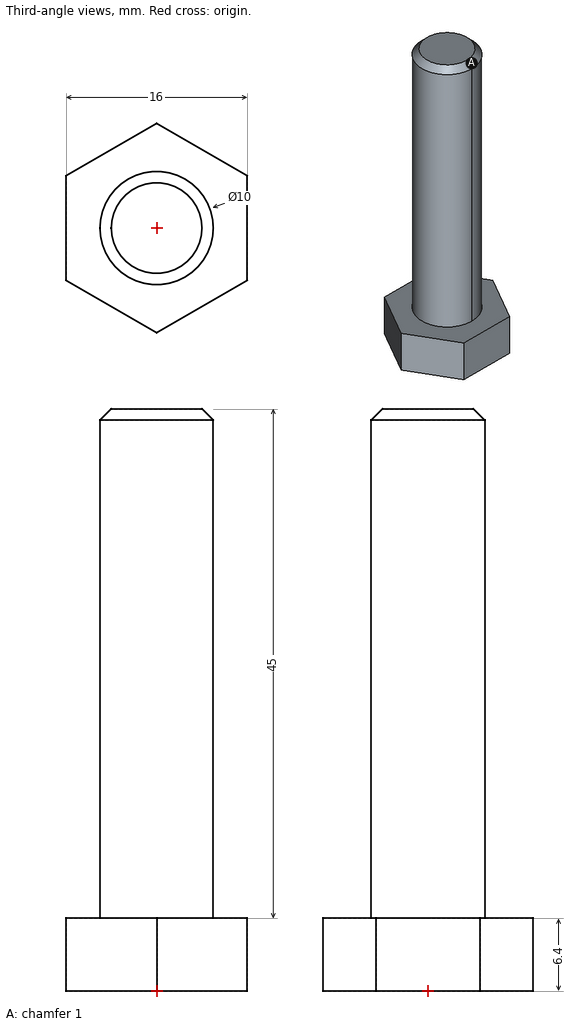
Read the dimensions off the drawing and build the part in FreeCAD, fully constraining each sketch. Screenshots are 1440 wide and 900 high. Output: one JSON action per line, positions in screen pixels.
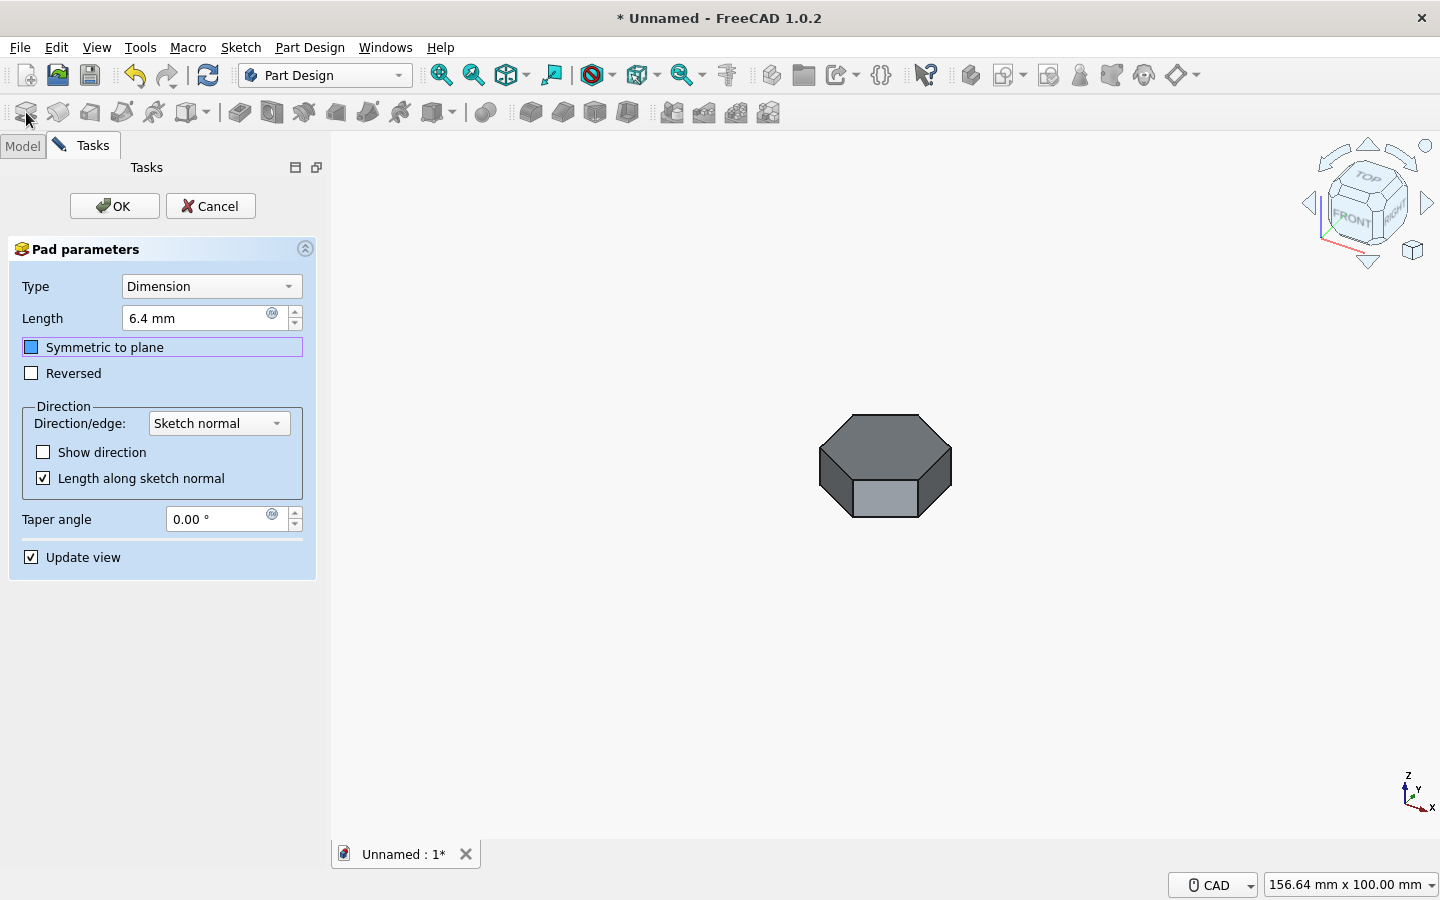
{"action": "left_click", "coordinate": [115, 206]}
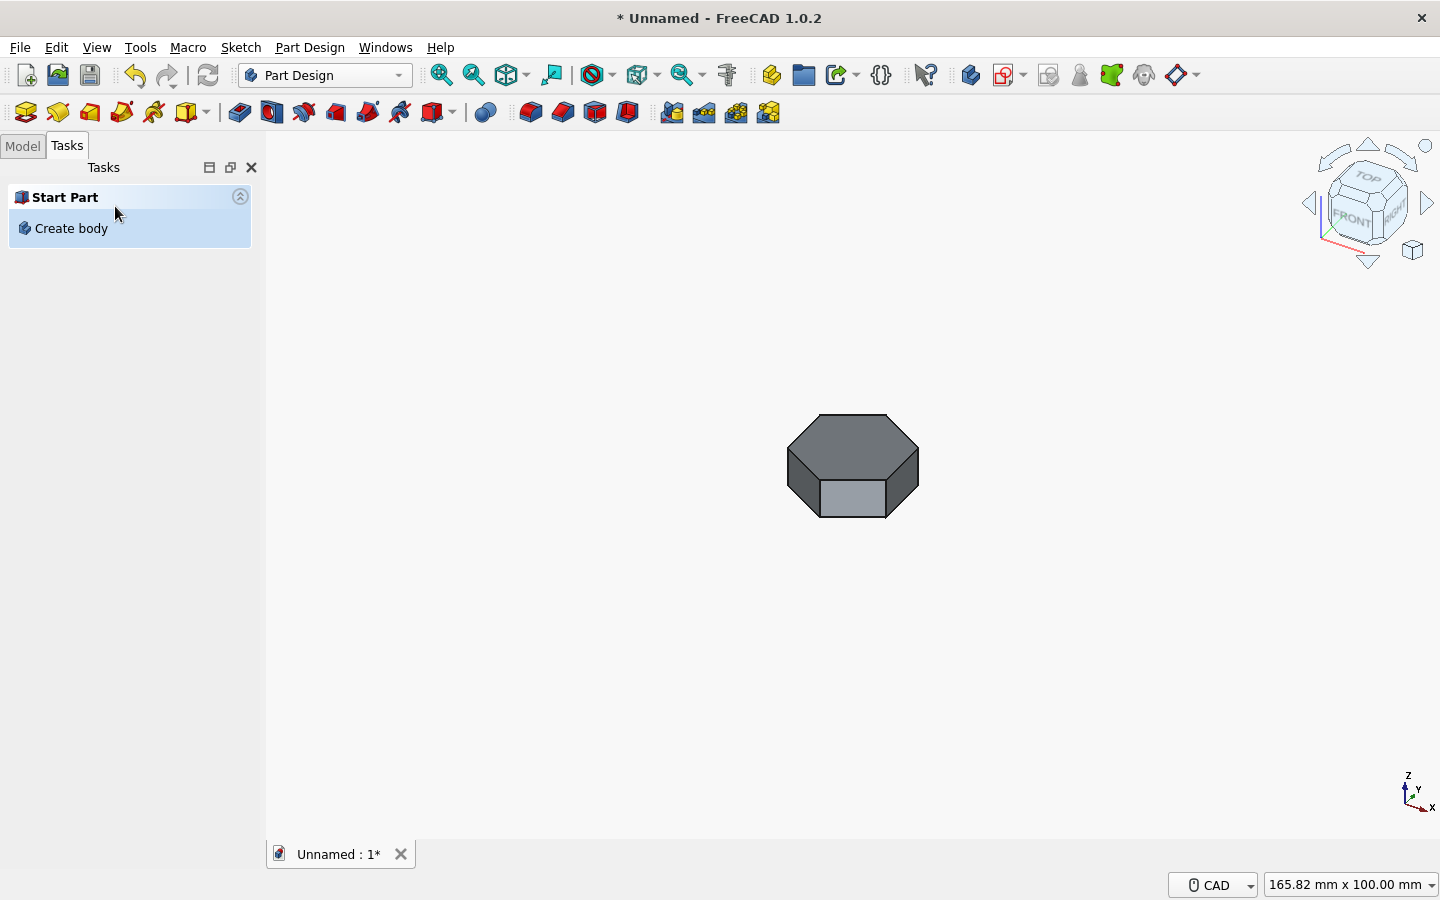
{"action": "left_click", "coordinate": [442, 76]}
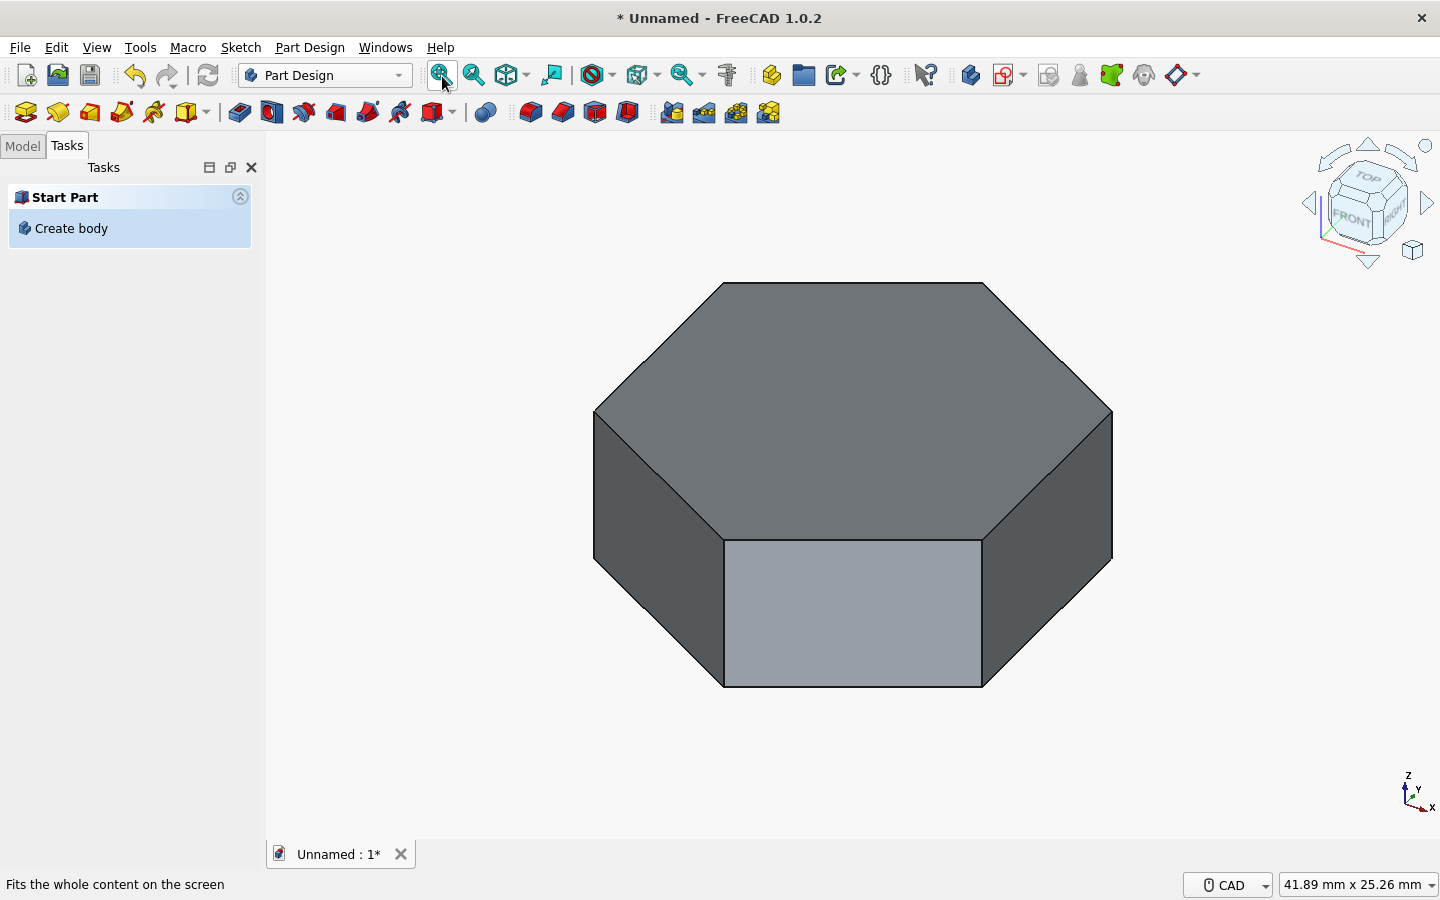
{"action": "left_click", "coordinate": [853, 411]}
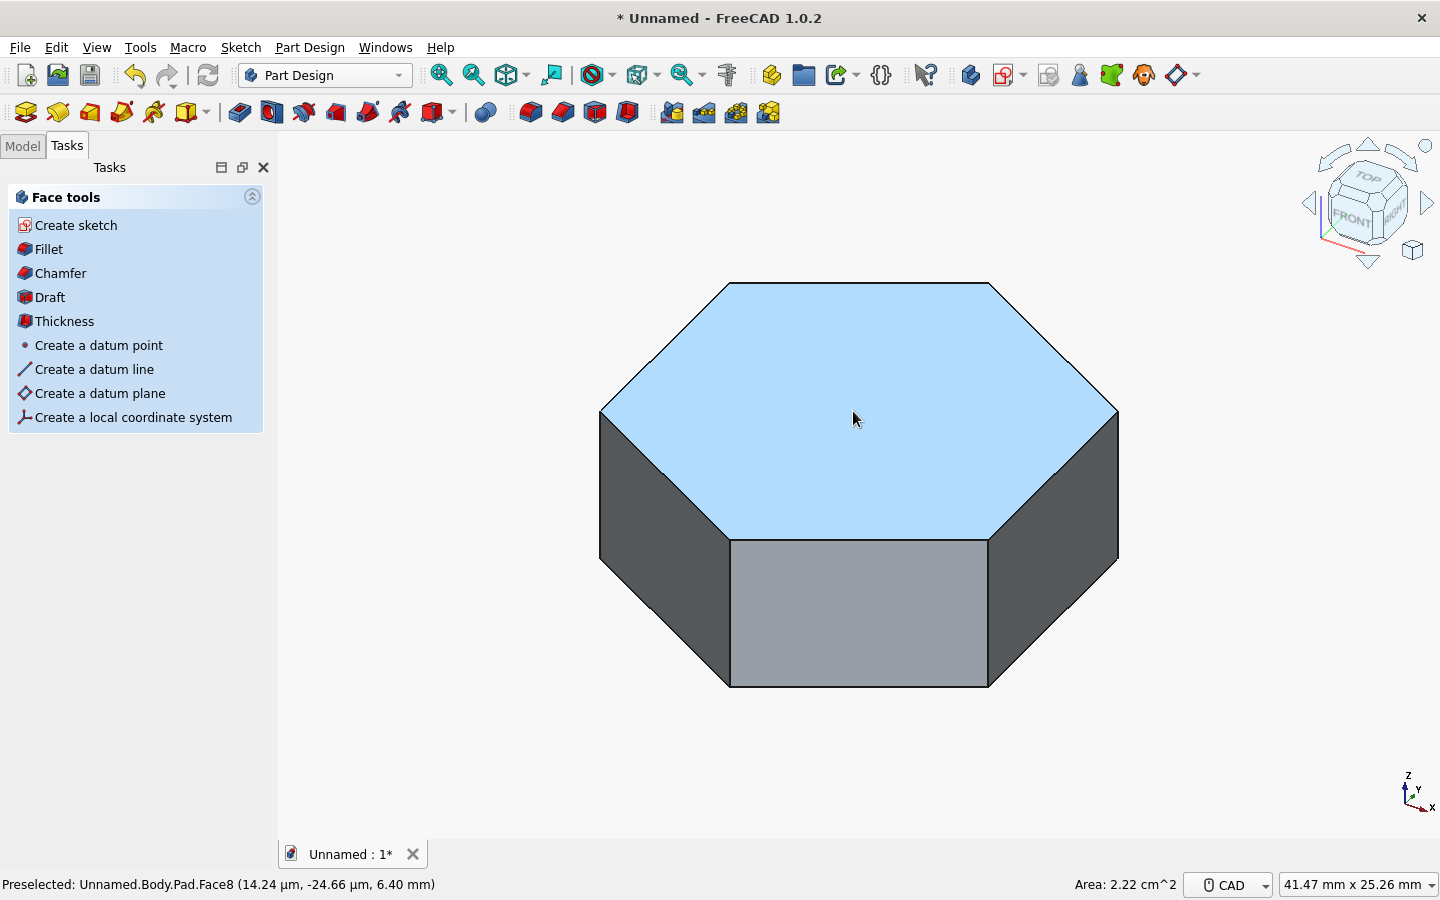
{"action": "left_click", "coordinate": [1004, 76]}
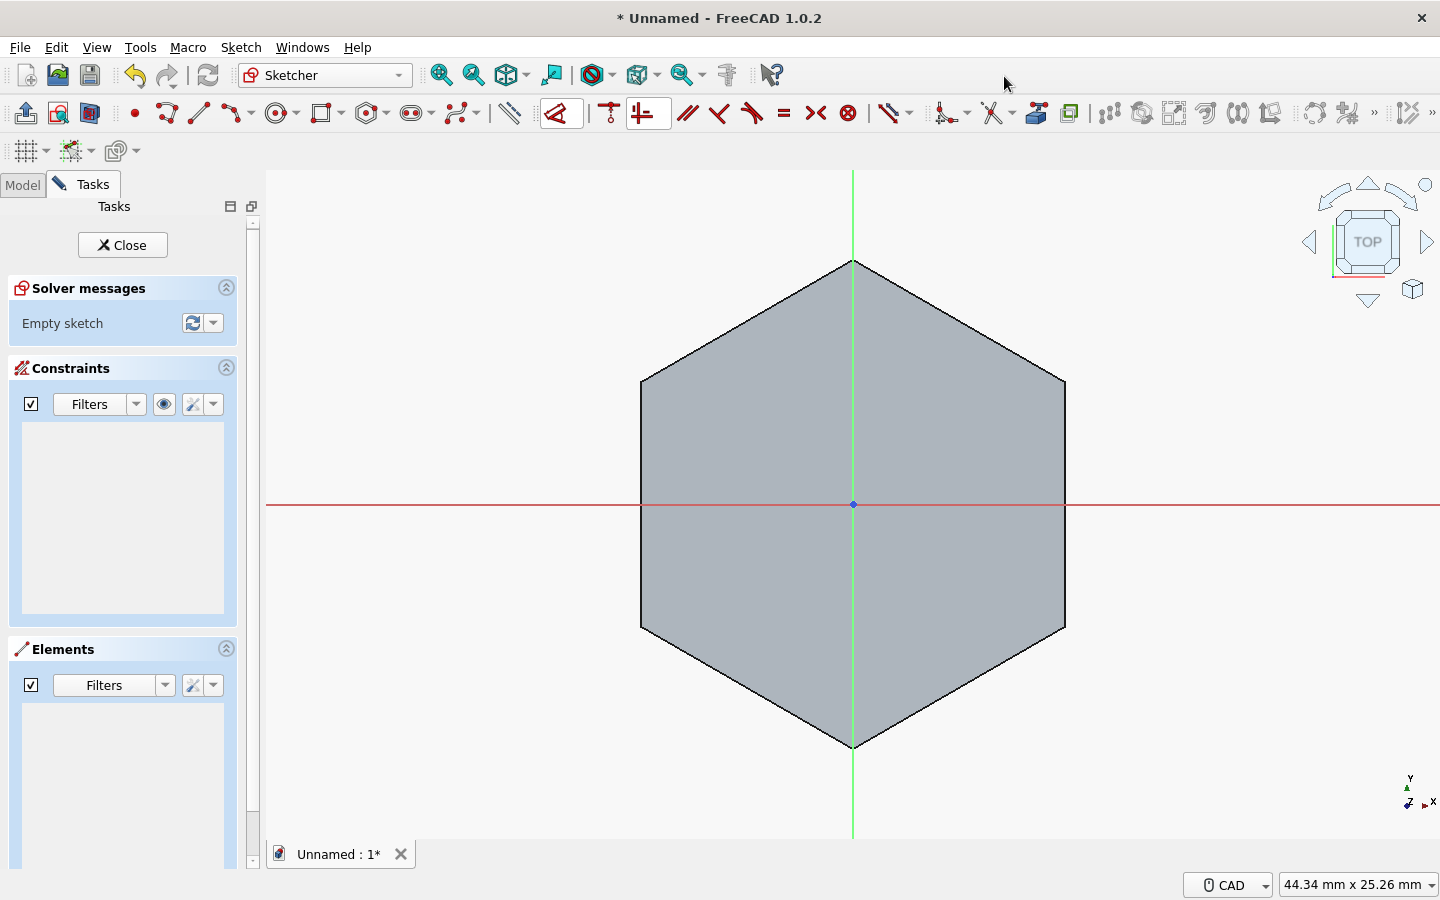
{"action": "scroll", "coordinate": [992, 504], "scroll_direction": "up", "scroll_amount": 2}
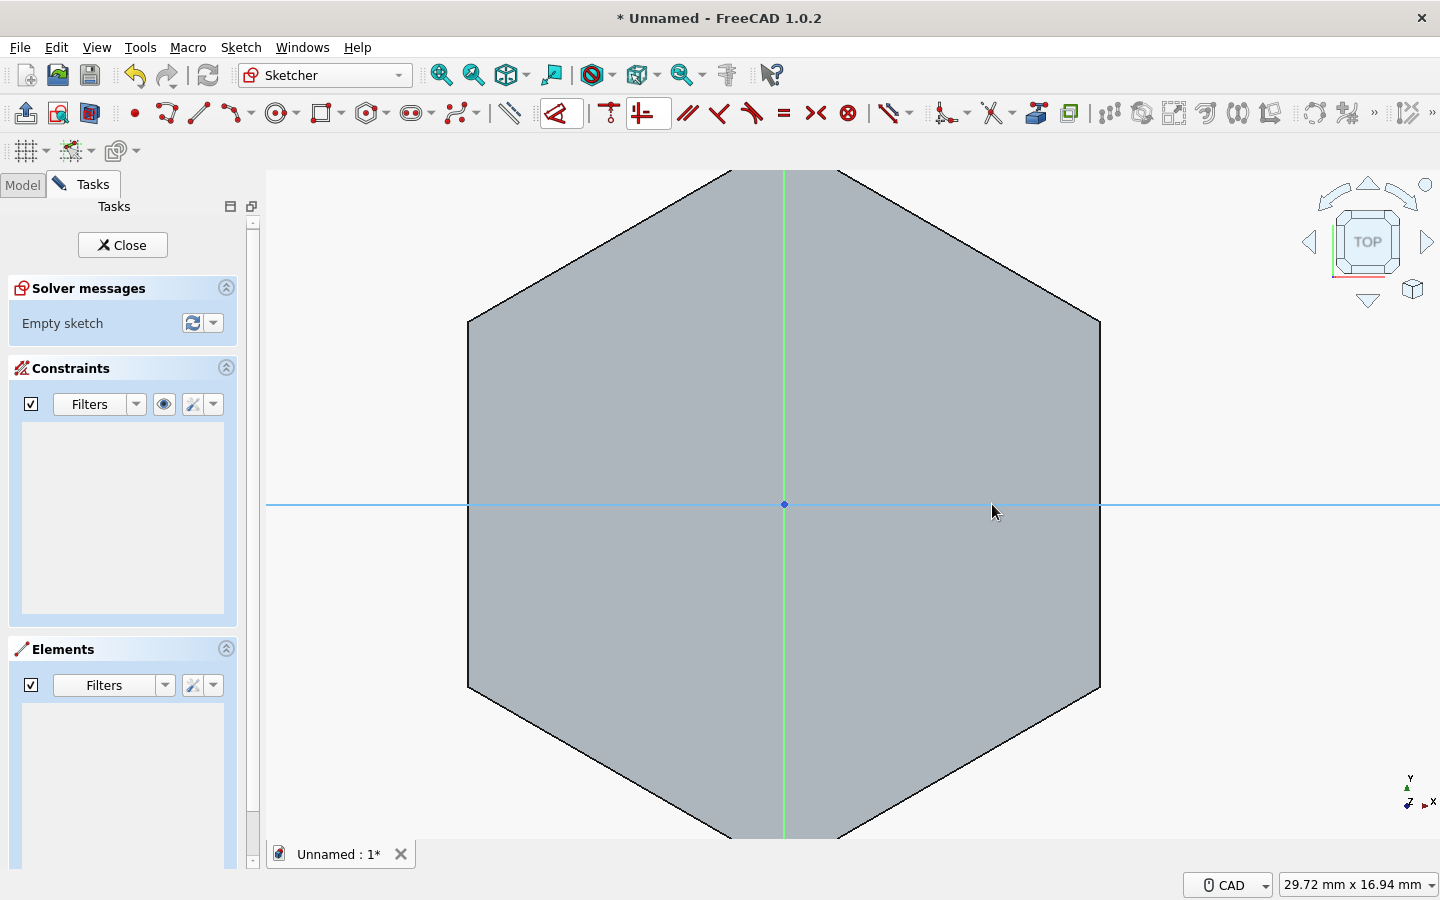
{"action": "left_click", "coordinate": [276, 114]}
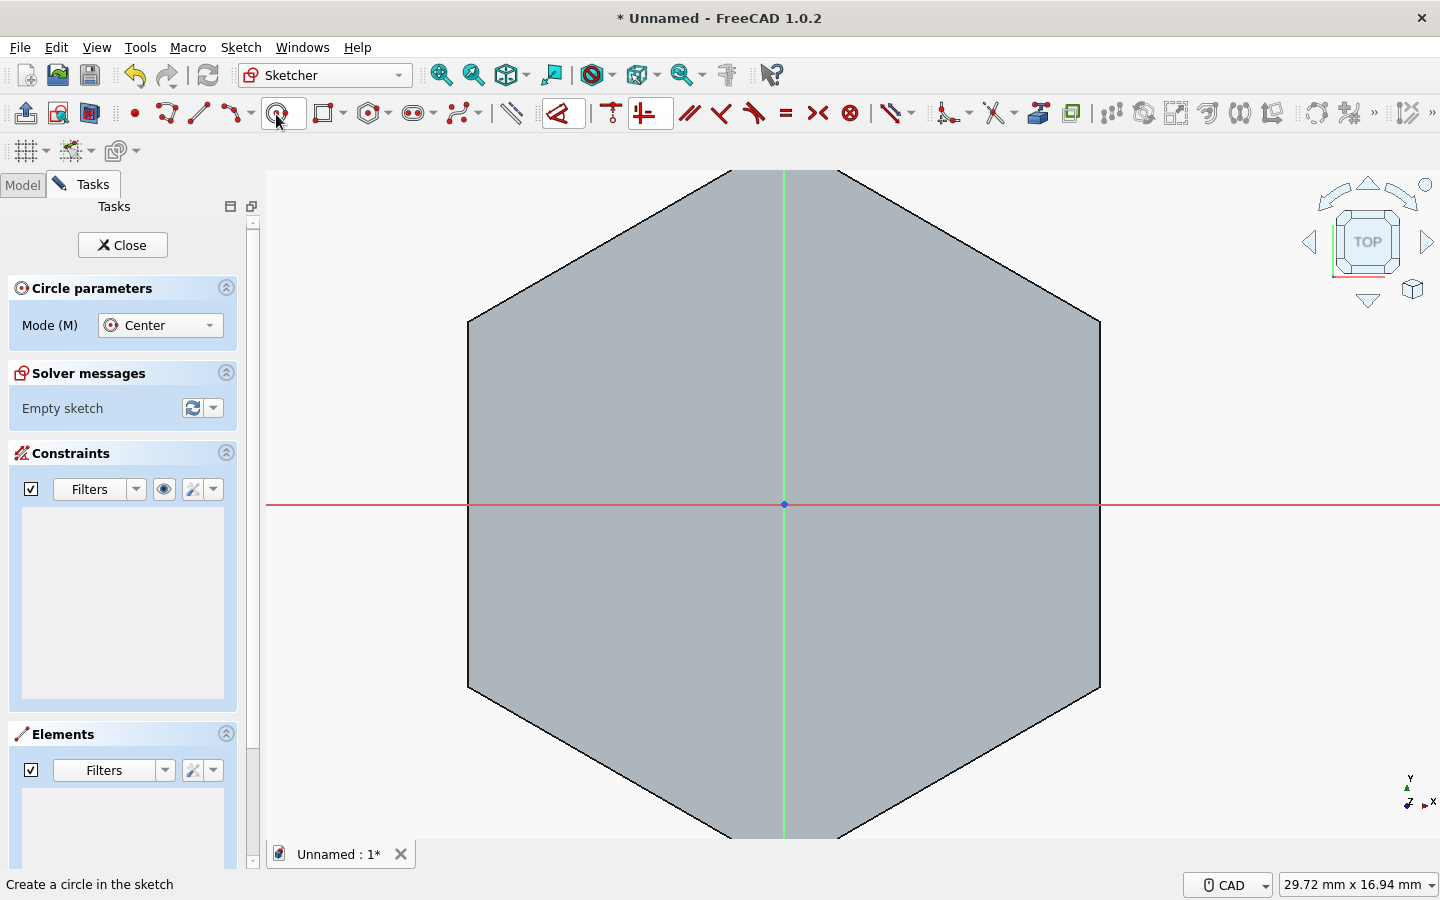
{"action": "left_click", "coordinate": [784, 504]}
{"action": "left_click", "coordinate": [924, 365]}
{"action": "key", "text": "Escape"}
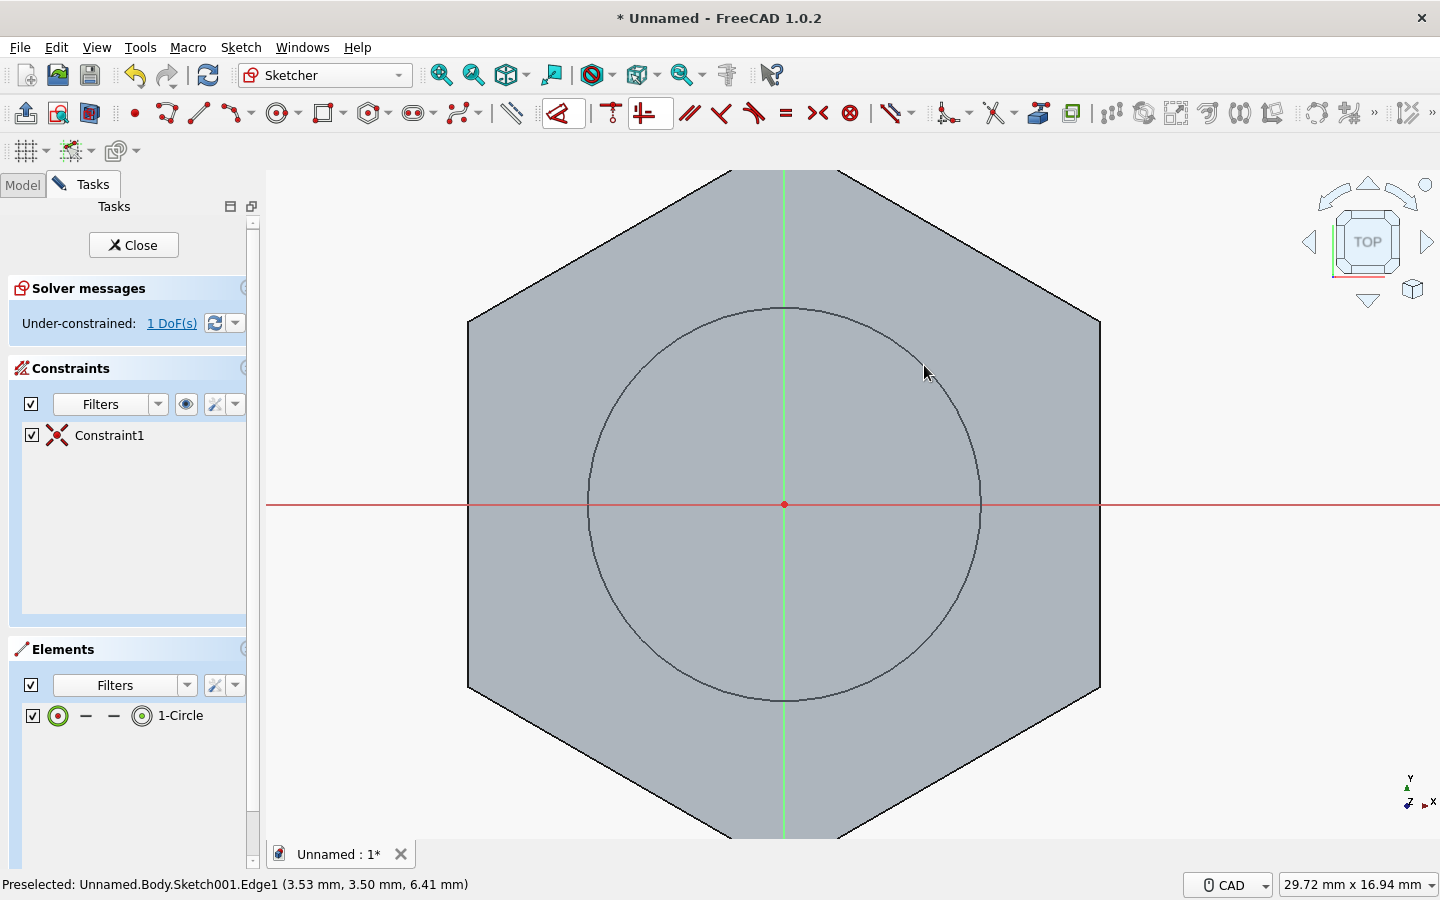
{"action": "left_click", "coordinate": [923, 365]}